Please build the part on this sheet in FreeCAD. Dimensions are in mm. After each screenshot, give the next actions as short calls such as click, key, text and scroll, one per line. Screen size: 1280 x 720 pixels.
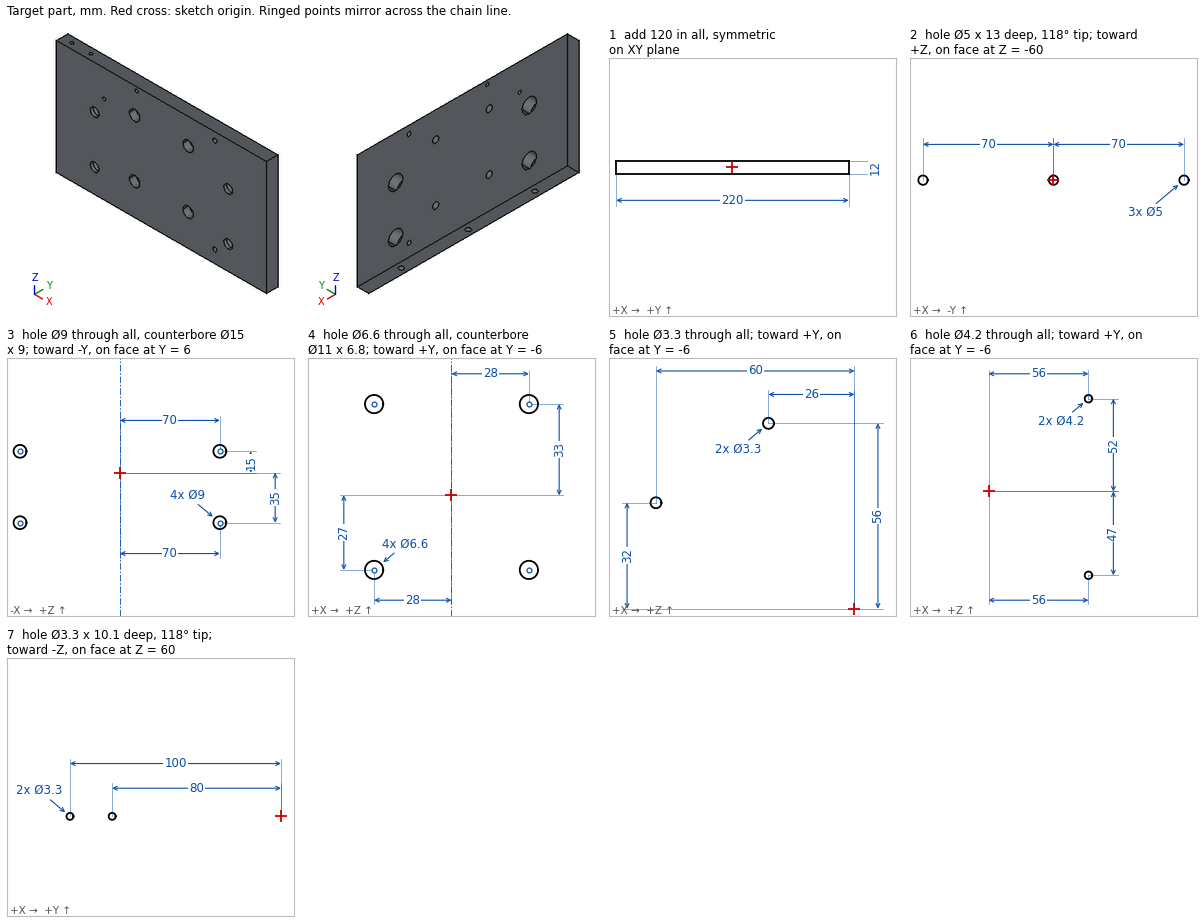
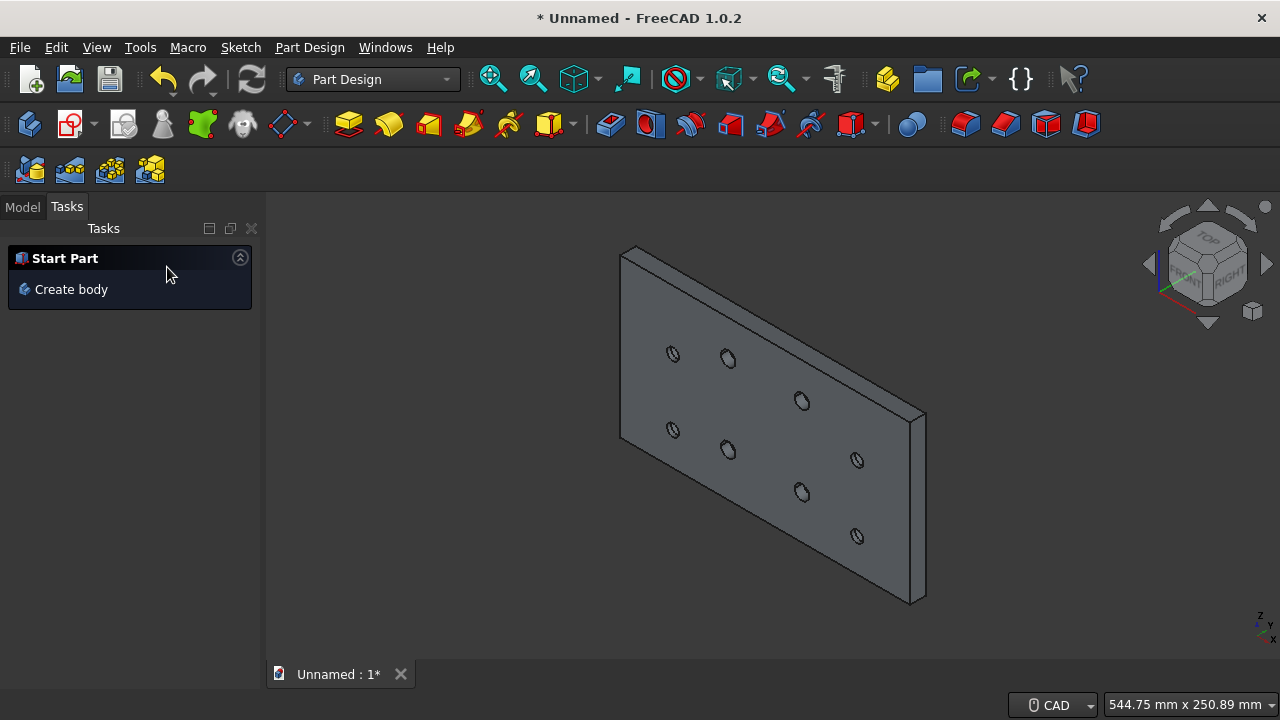
click(765, 429)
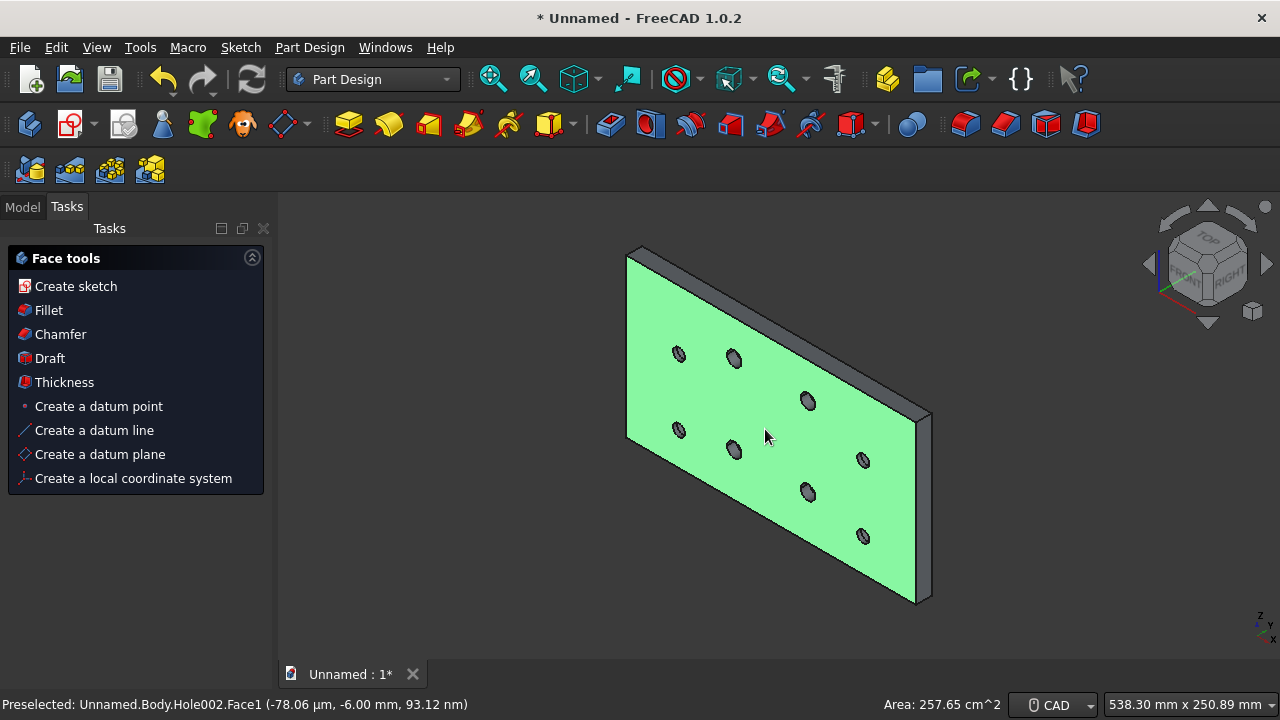
click(70, 124)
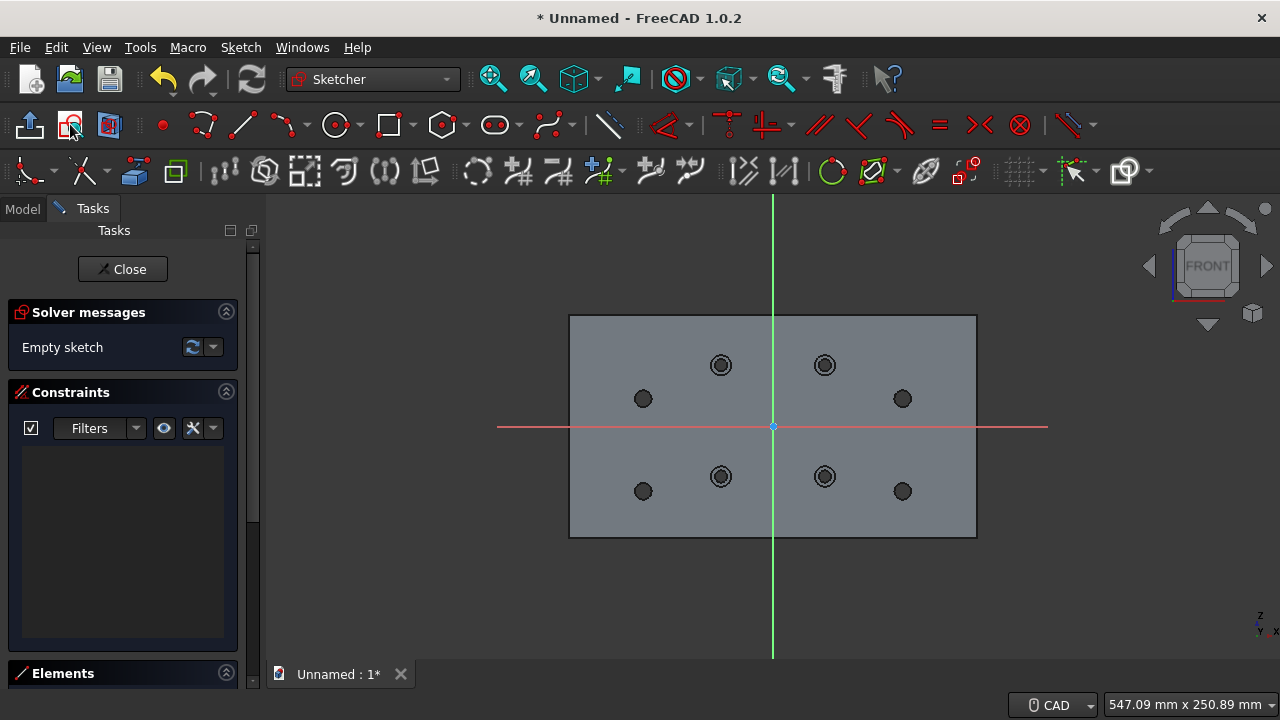
scroll(722, 342, up, 5)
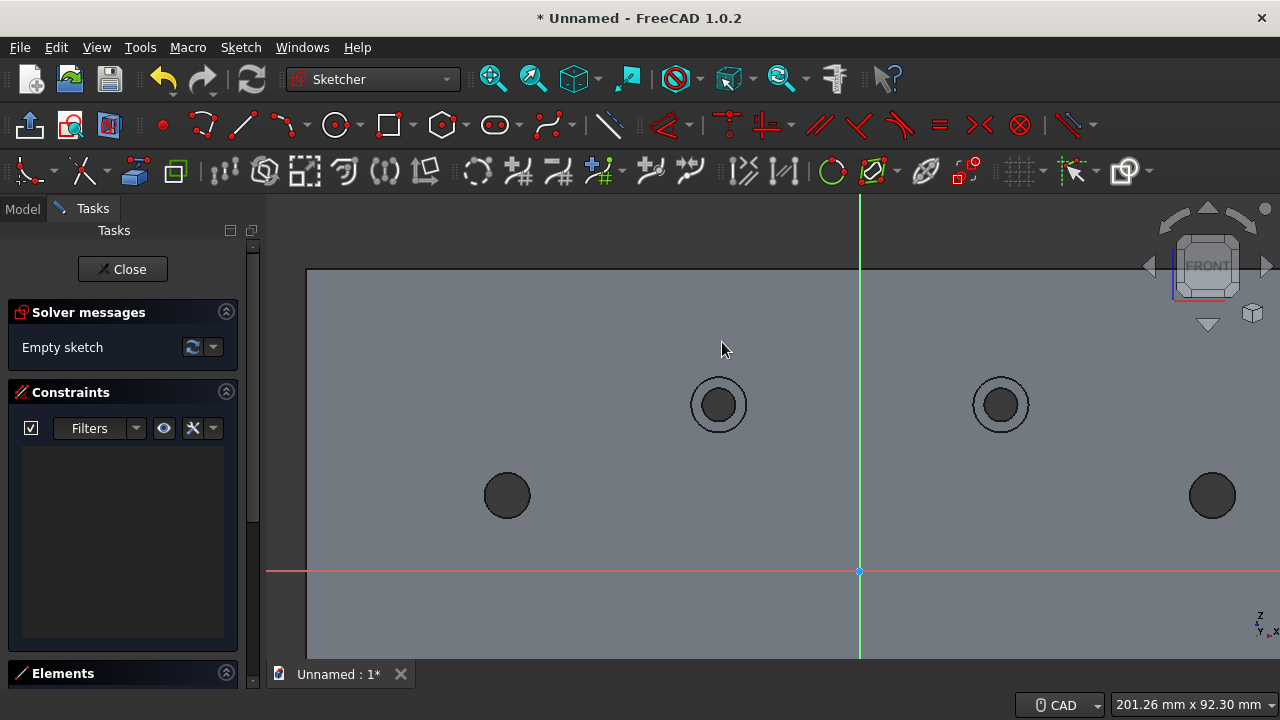
click(336, 126)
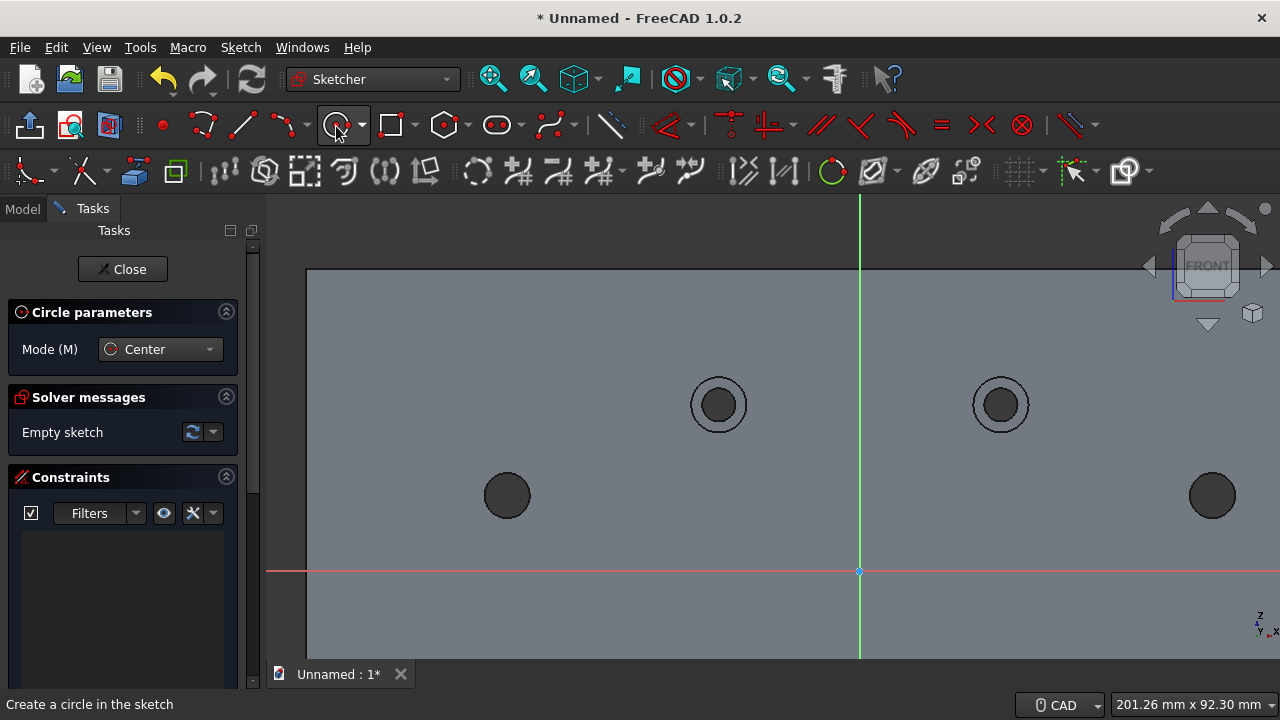
scroll(729, 289, up, 6)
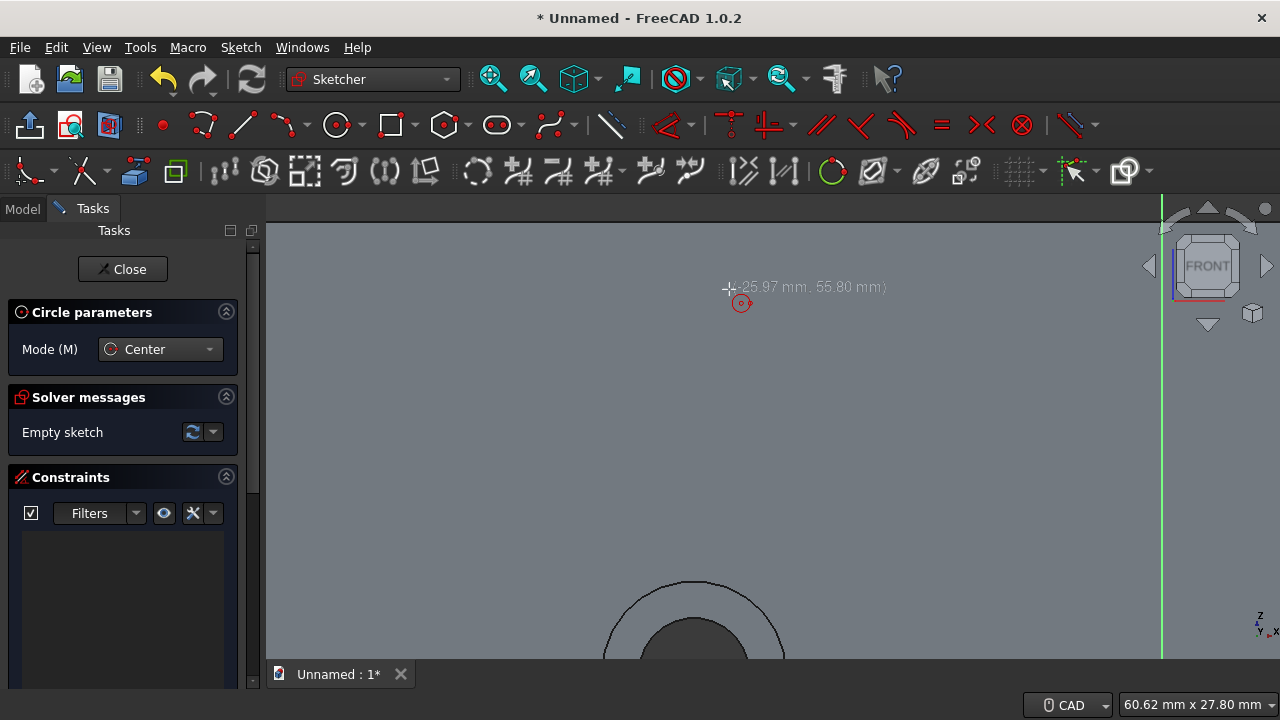
click(727, 289)
move(747, 269)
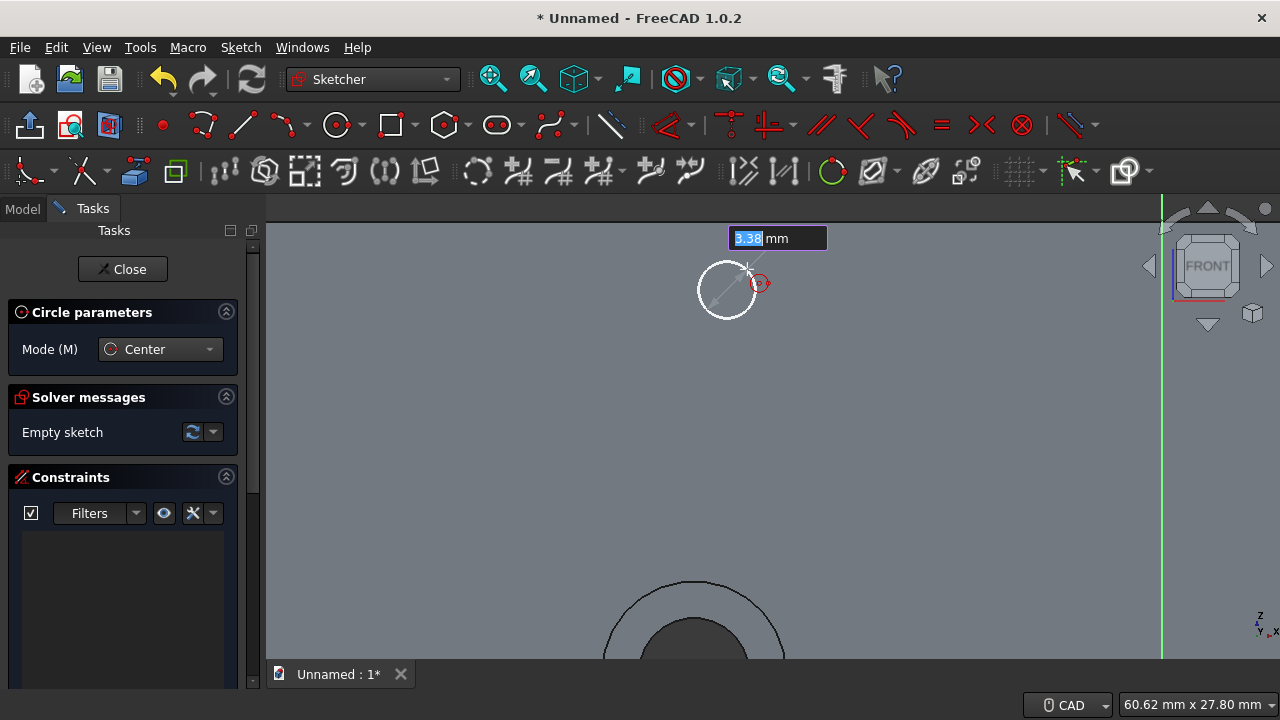
text(3.3)
key(Return)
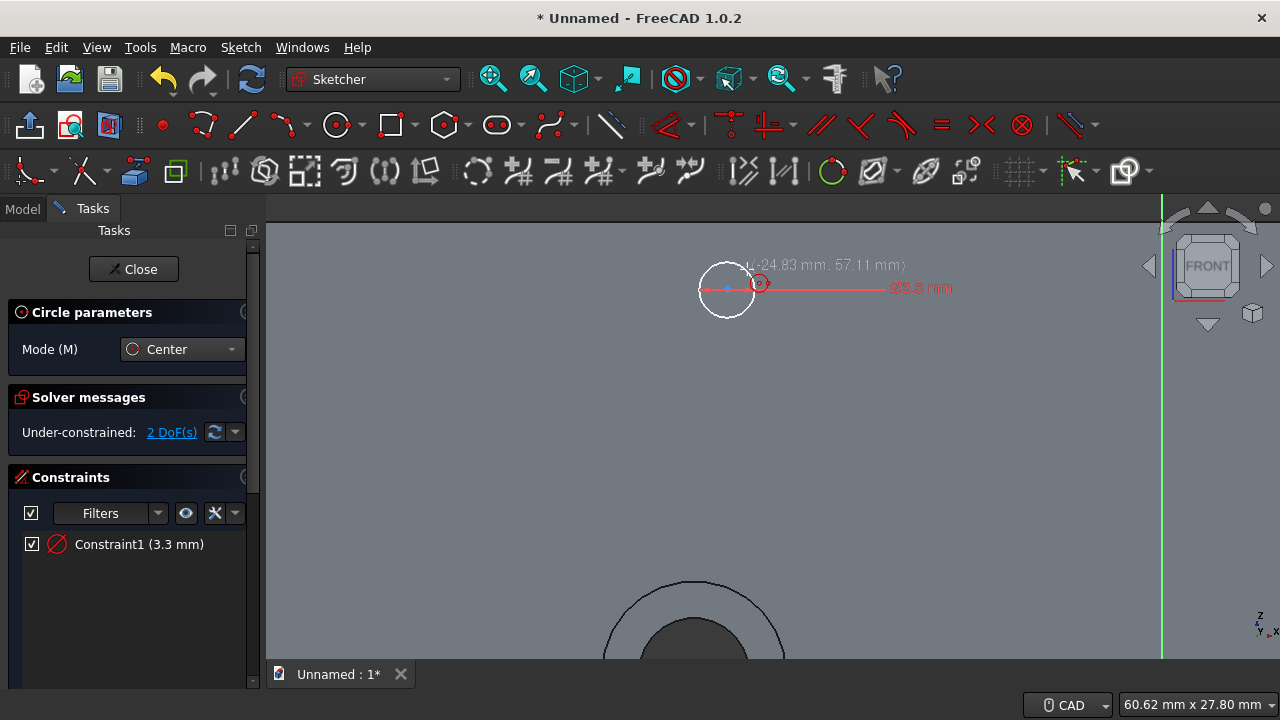
scroll(729, 290, down, 6)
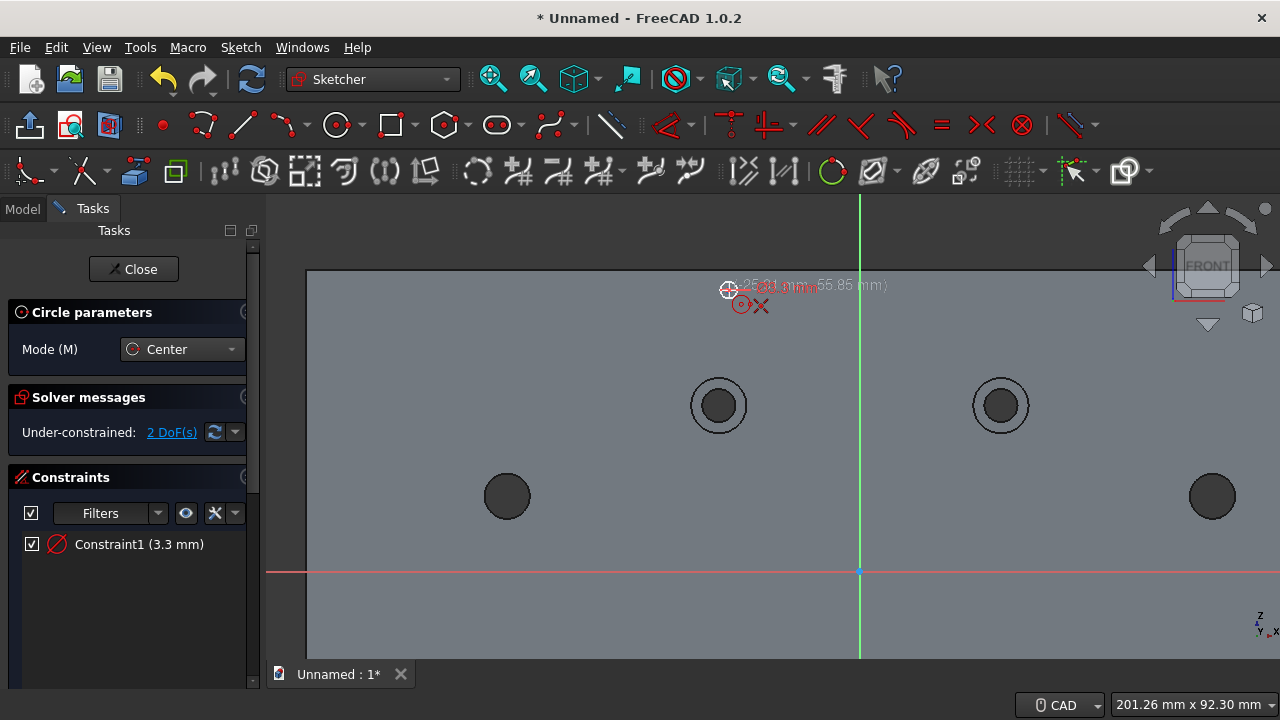
scroll(558, 411, up, 6)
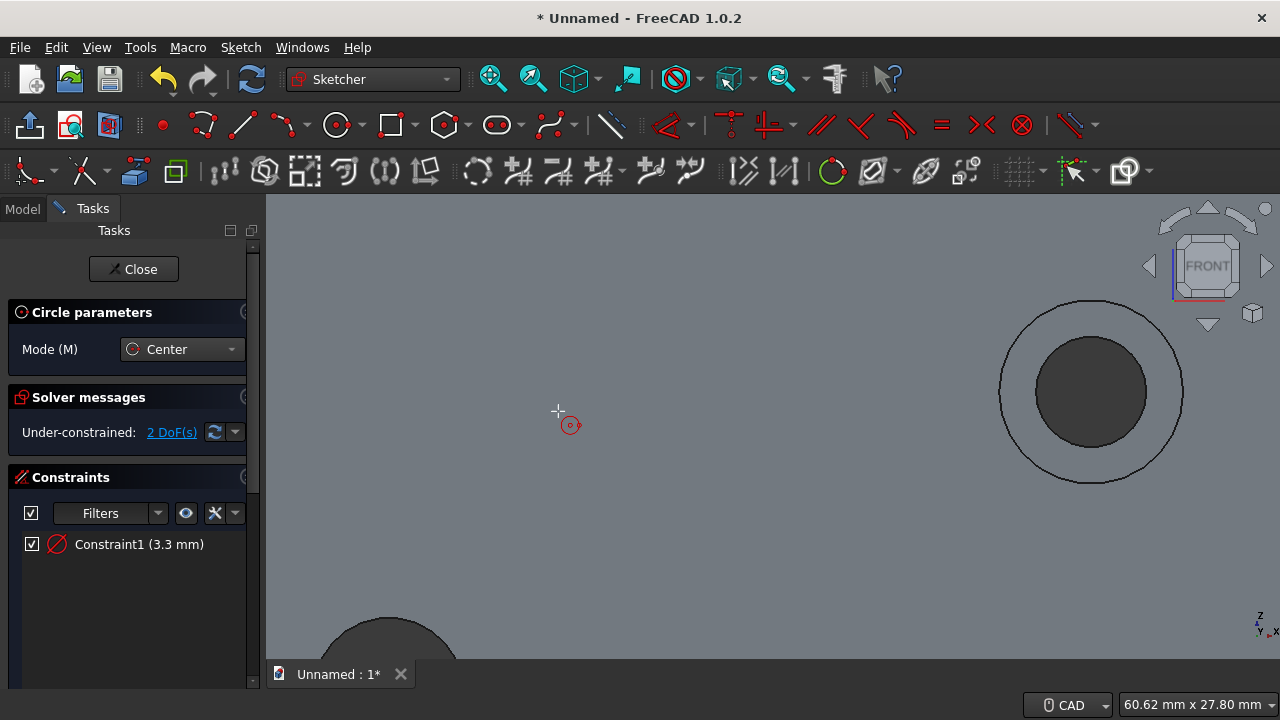
click(556, 409)
move(575, 389)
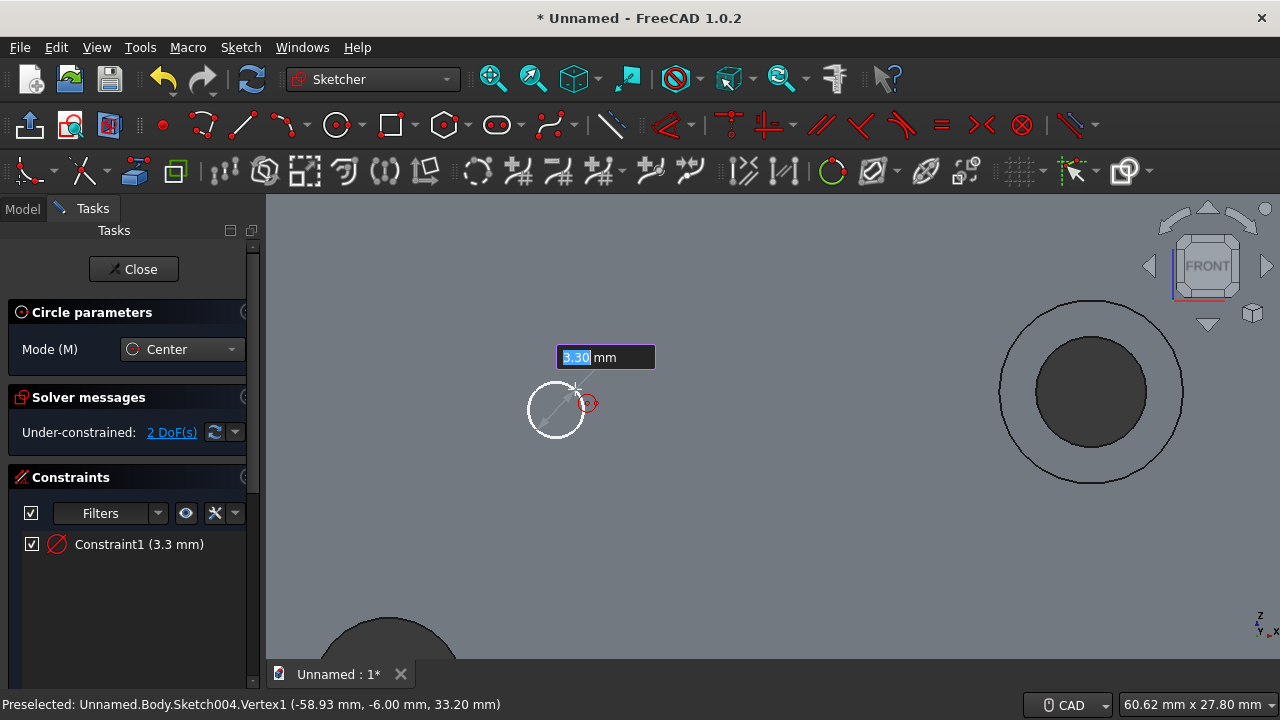
text(3.3)
key(Return)
key(Escape)